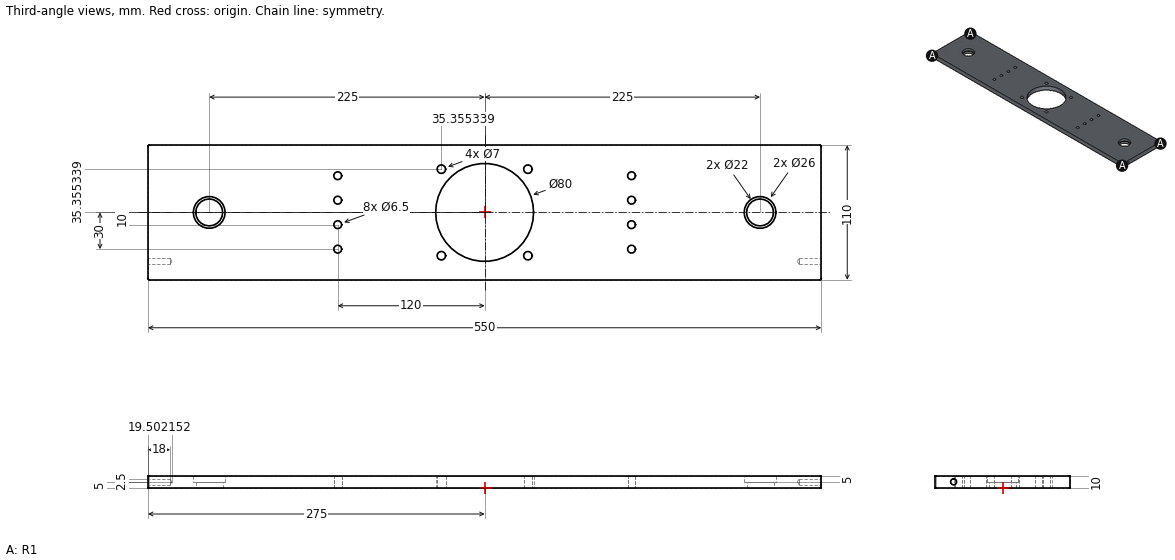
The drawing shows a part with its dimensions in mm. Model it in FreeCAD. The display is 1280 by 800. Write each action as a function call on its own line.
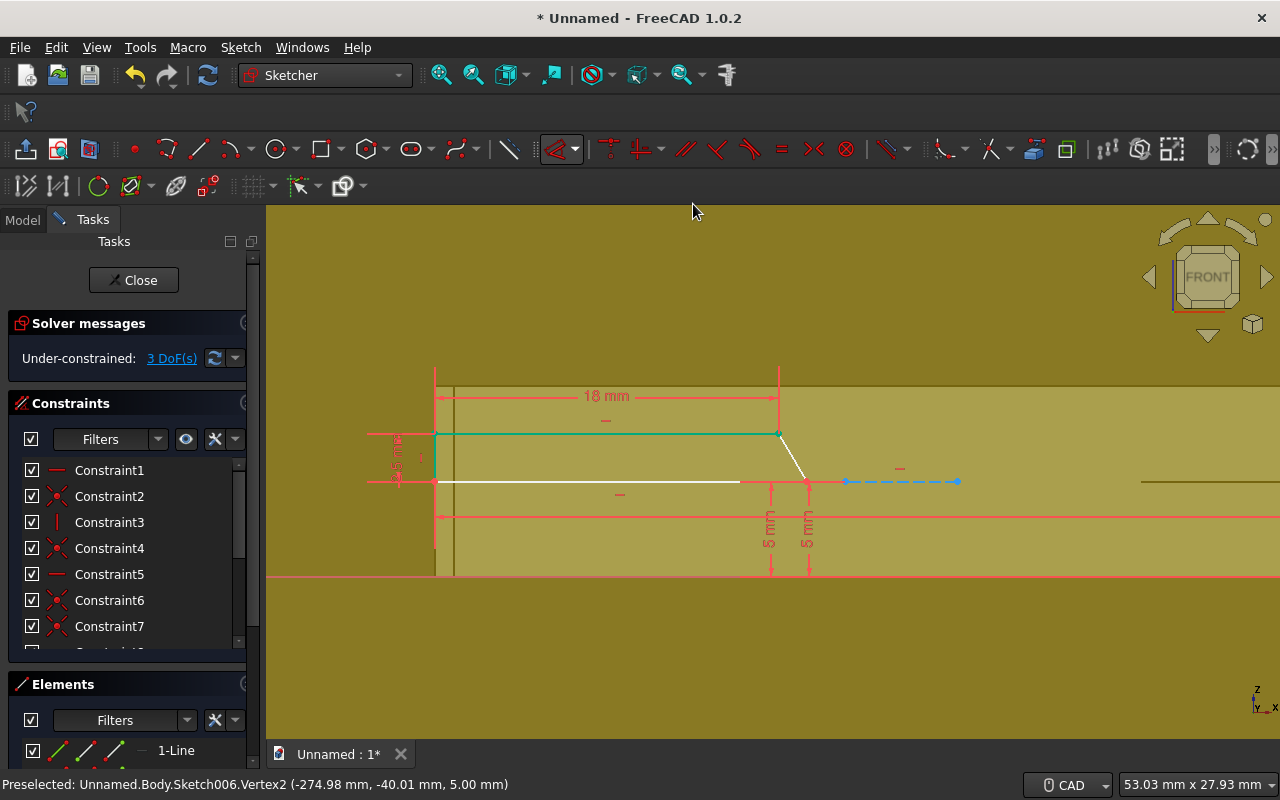
click(695, 482)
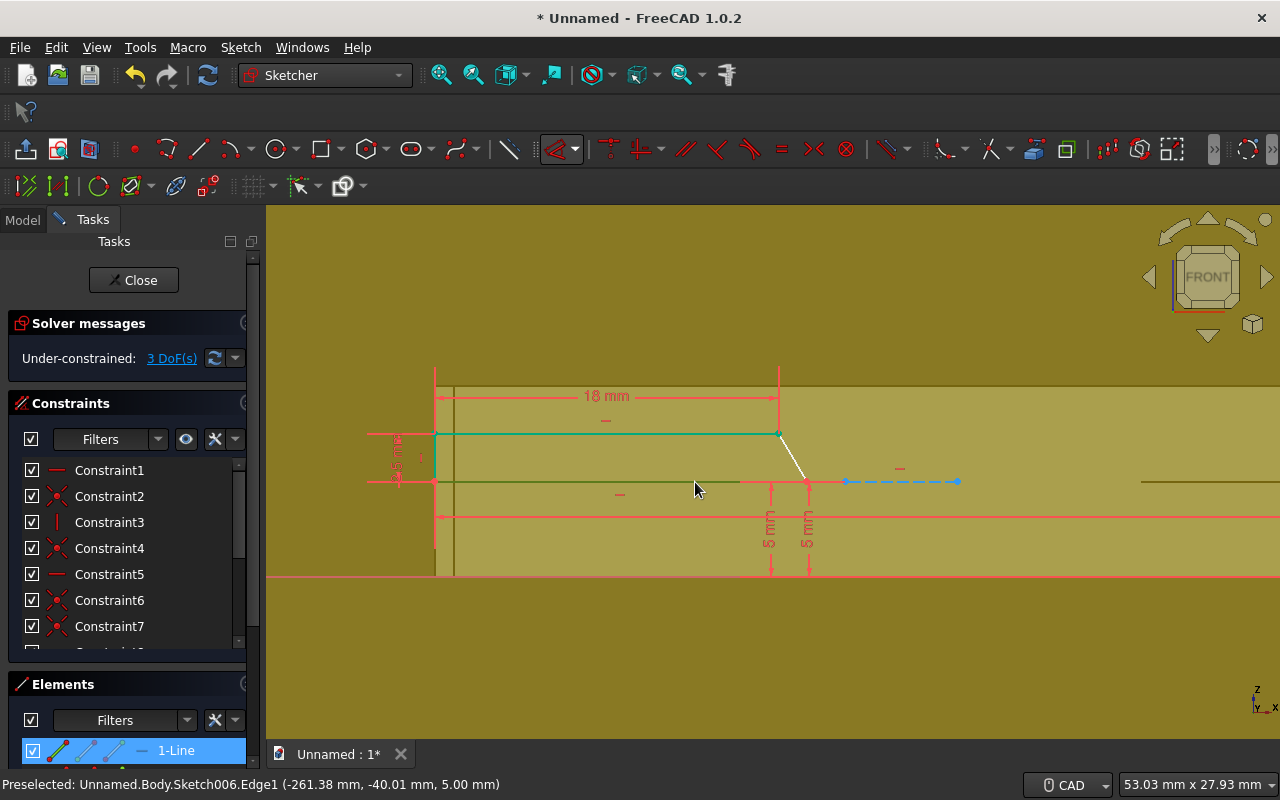
key(l)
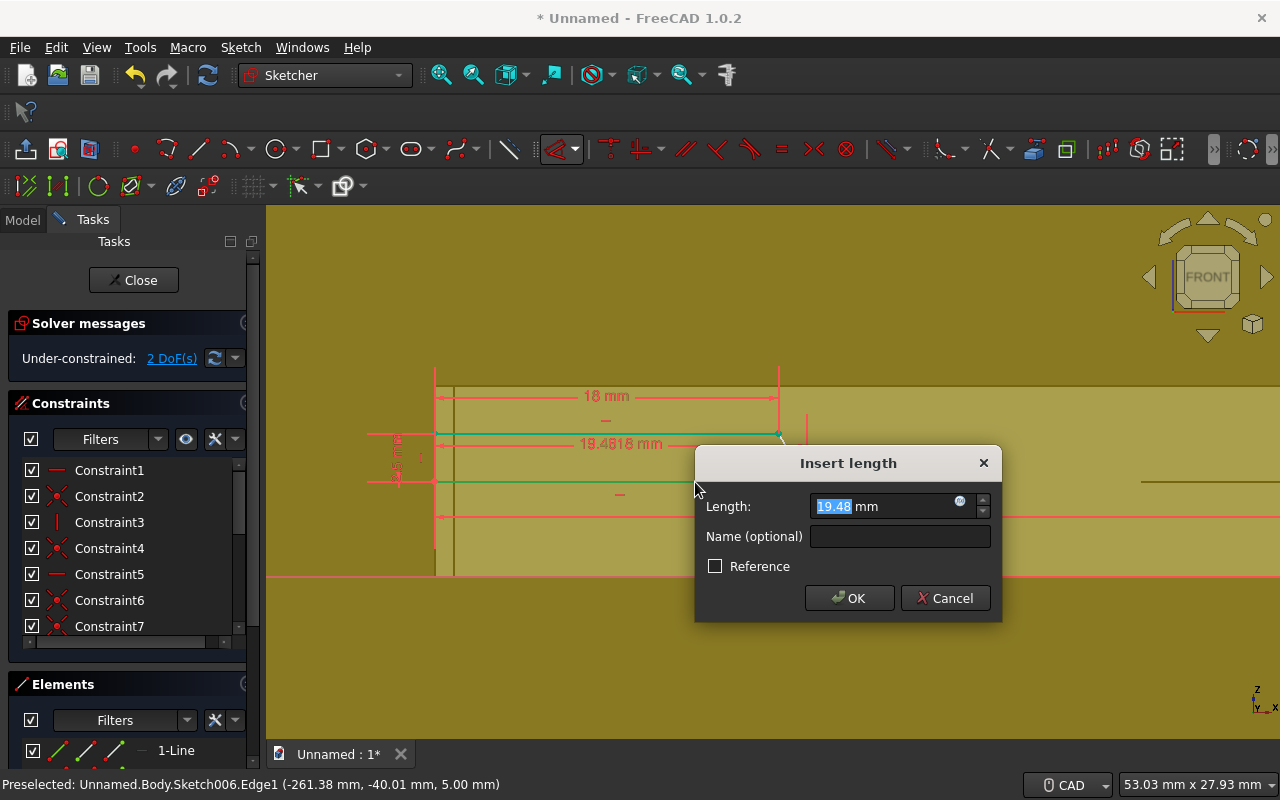
text(19.502152)
key(Return)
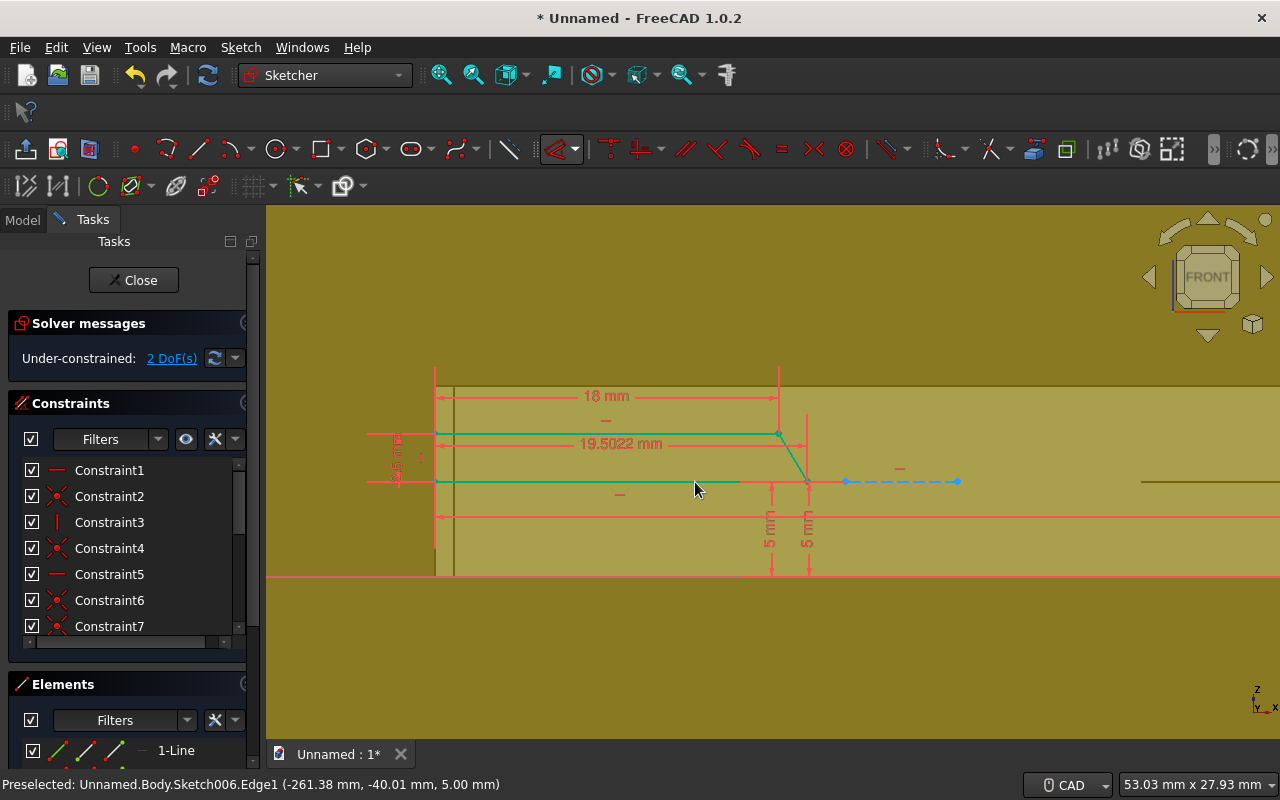
click(134, 280)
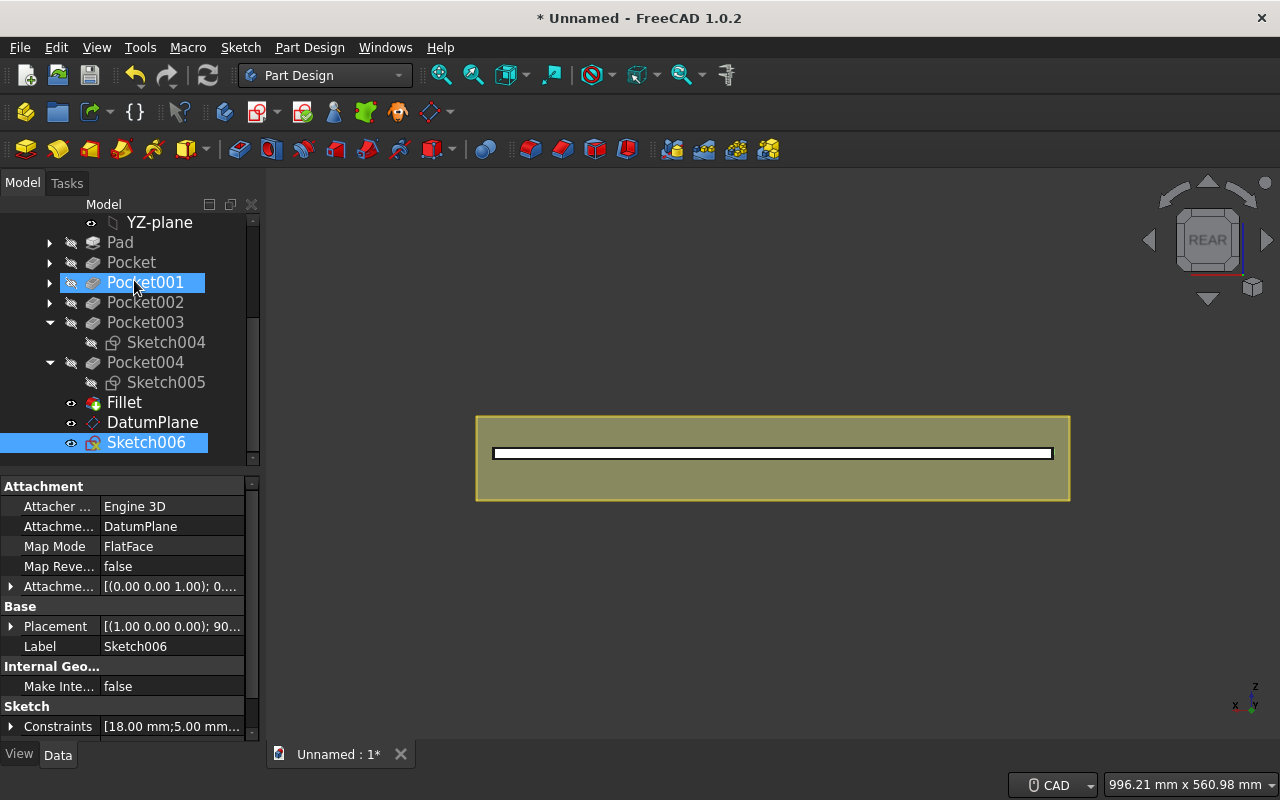
click(304, 150)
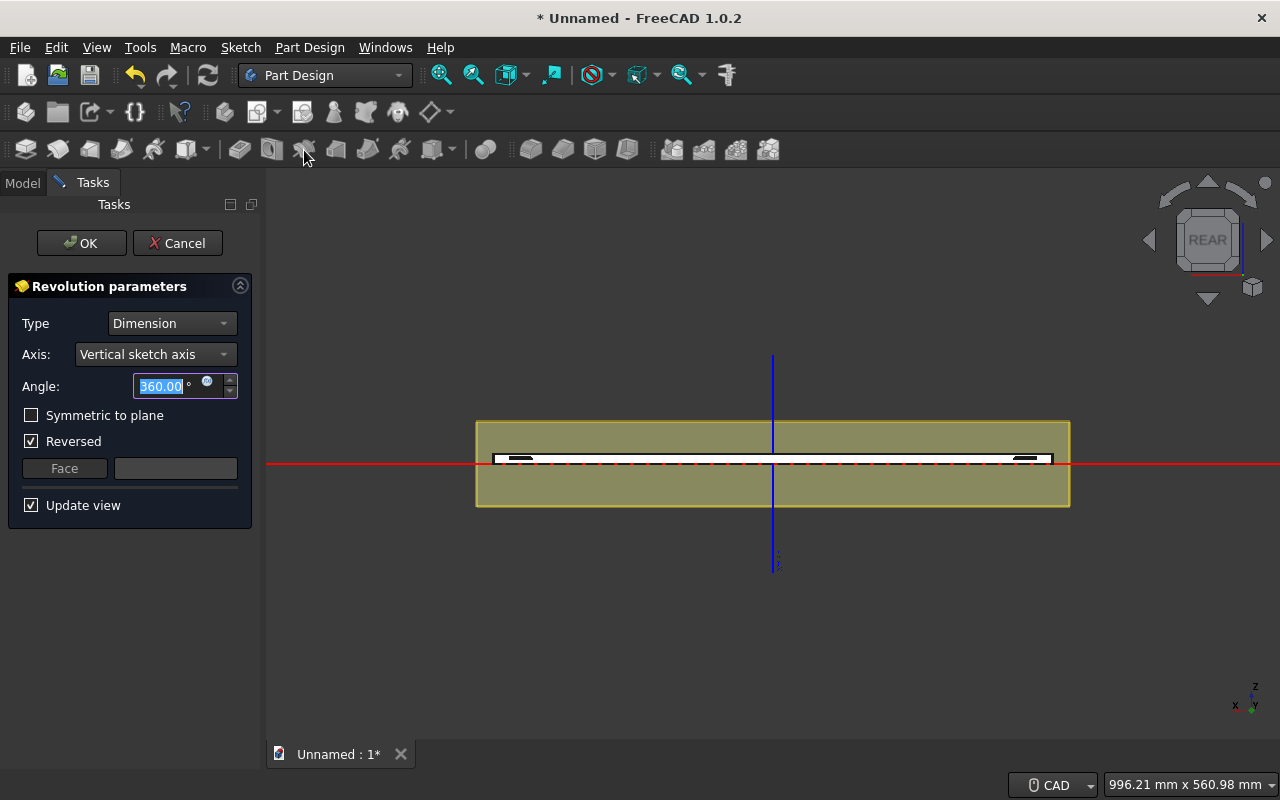
click(156, 354)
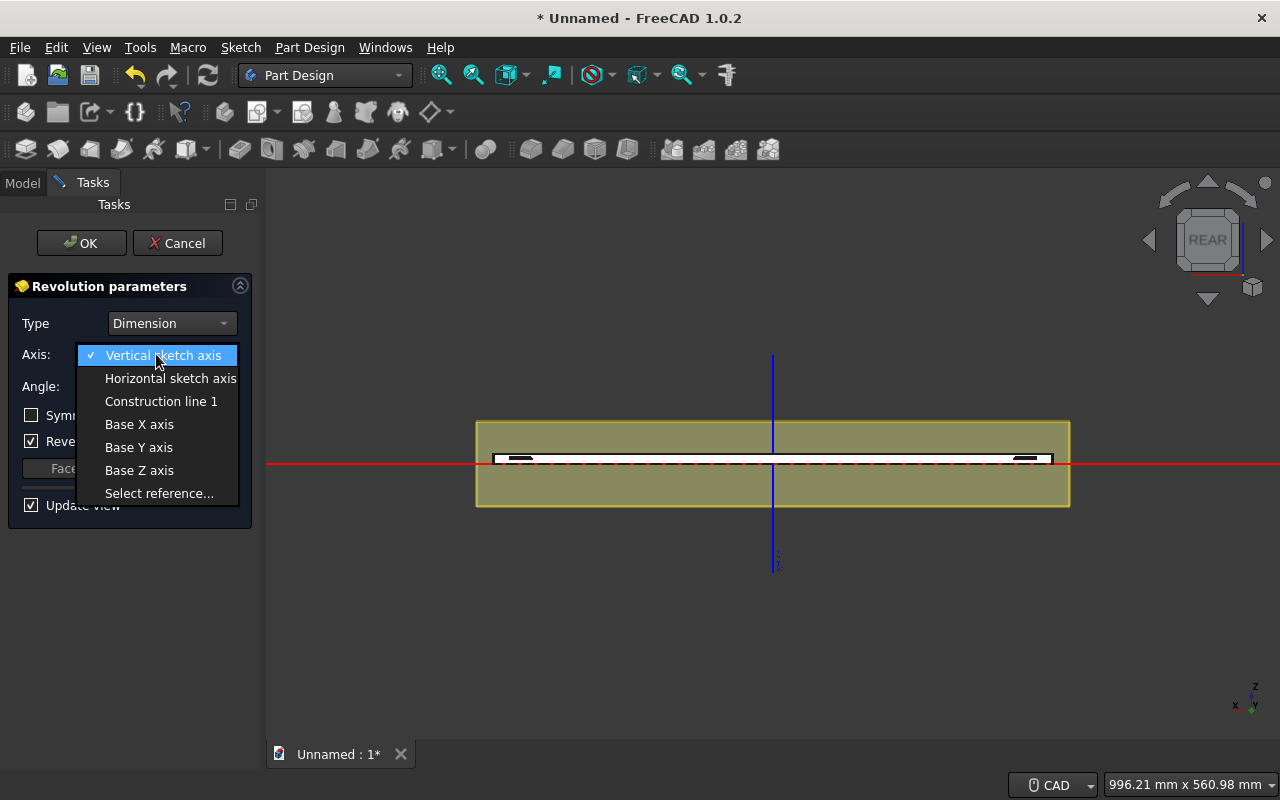
click(156, 402)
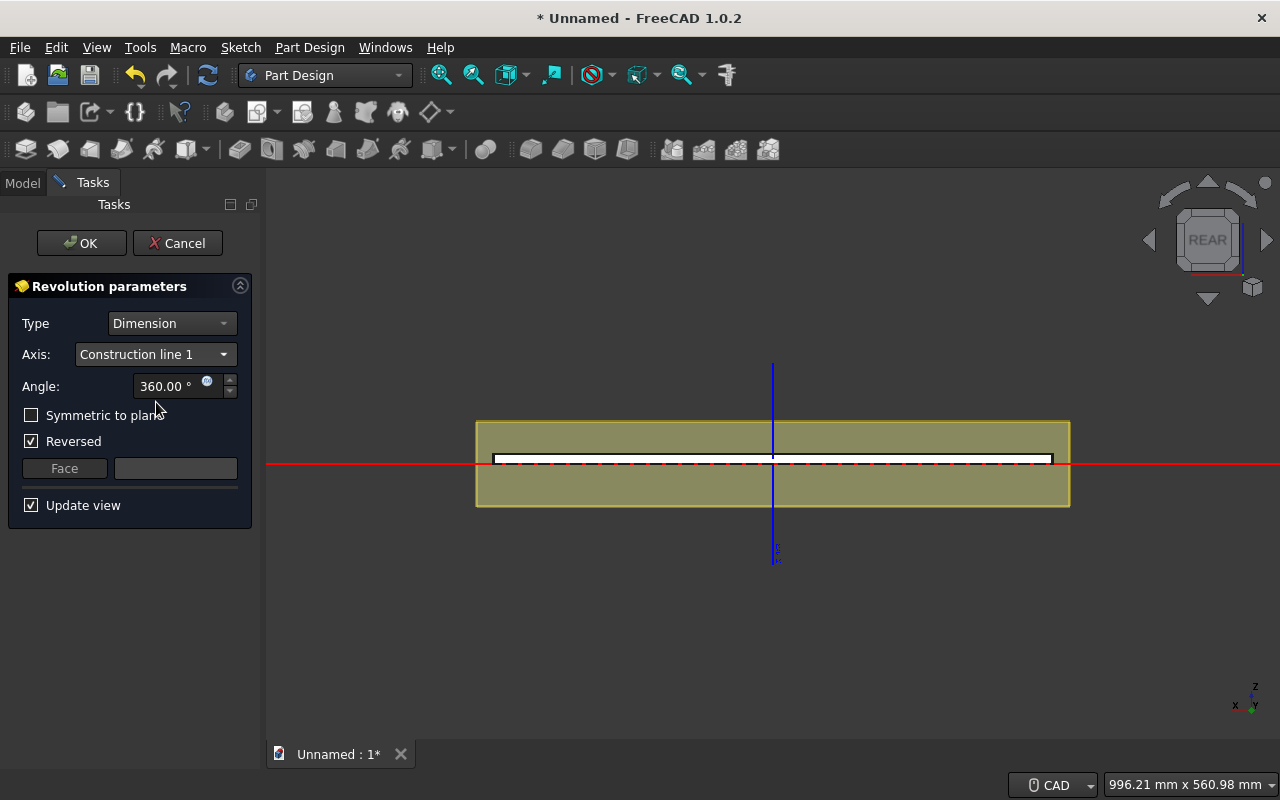
click(82, 243)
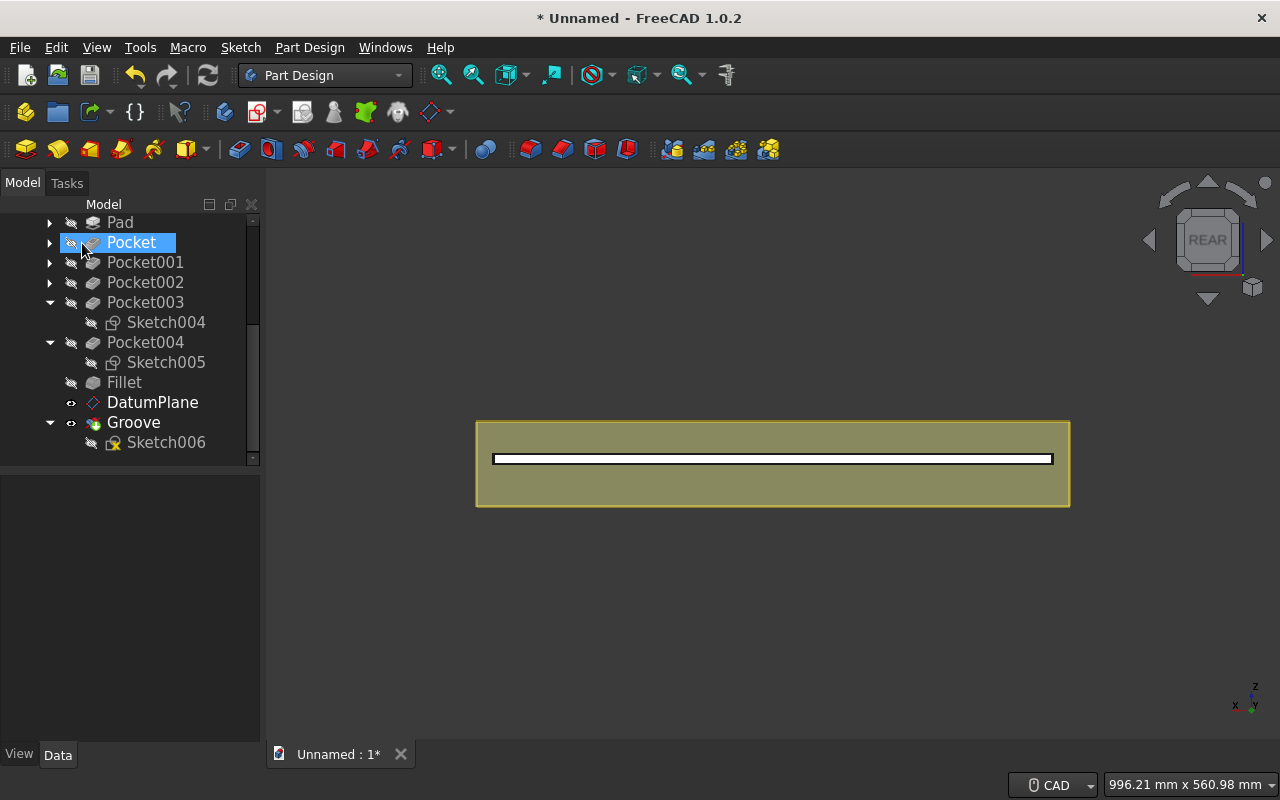
click(116, 403)
key(space)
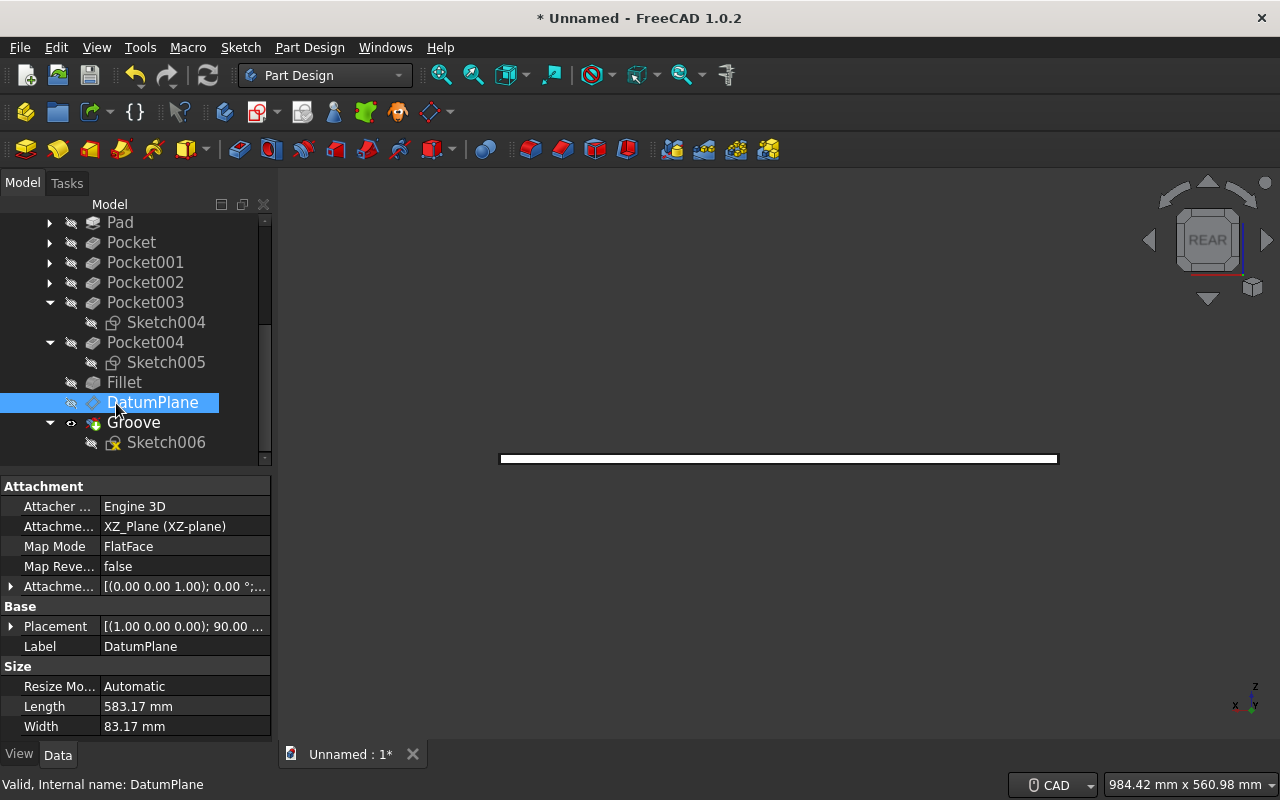
click(116, 423)